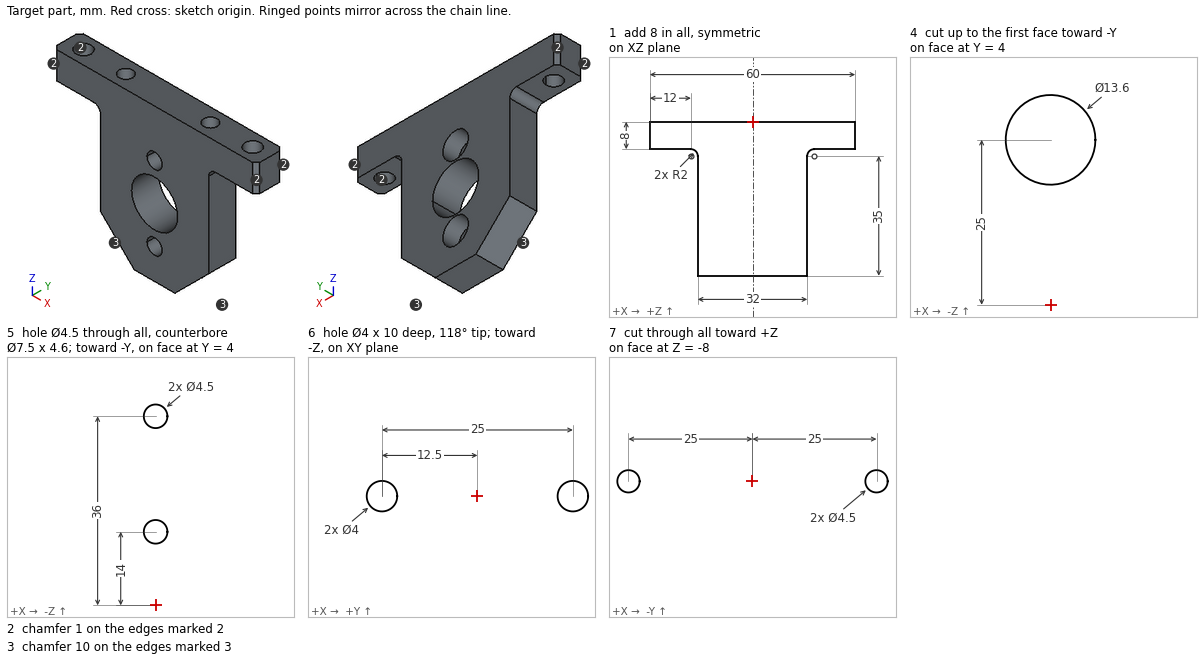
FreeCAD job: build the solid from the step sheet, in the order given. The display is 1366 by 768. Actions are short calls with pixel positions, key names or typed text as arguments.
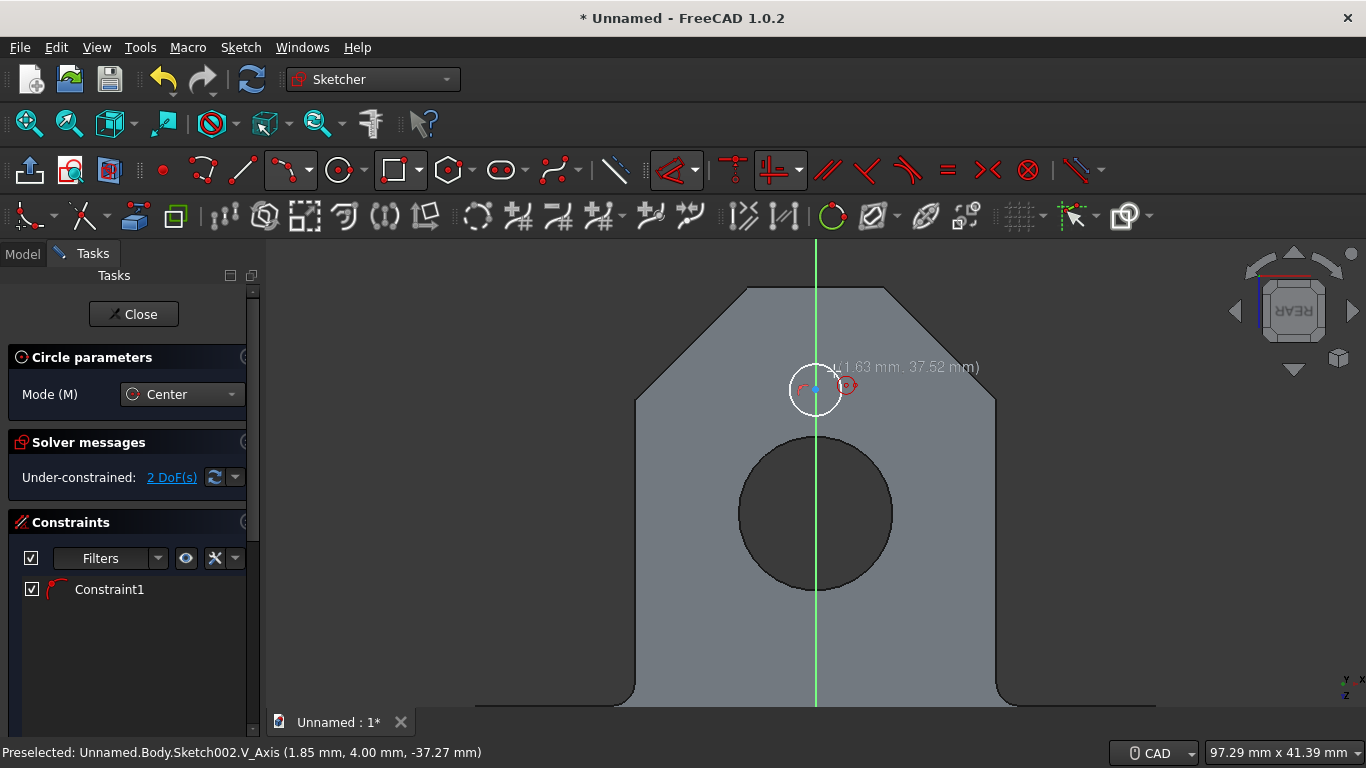
click(816, 638)
click(834, 620)
key(Escape)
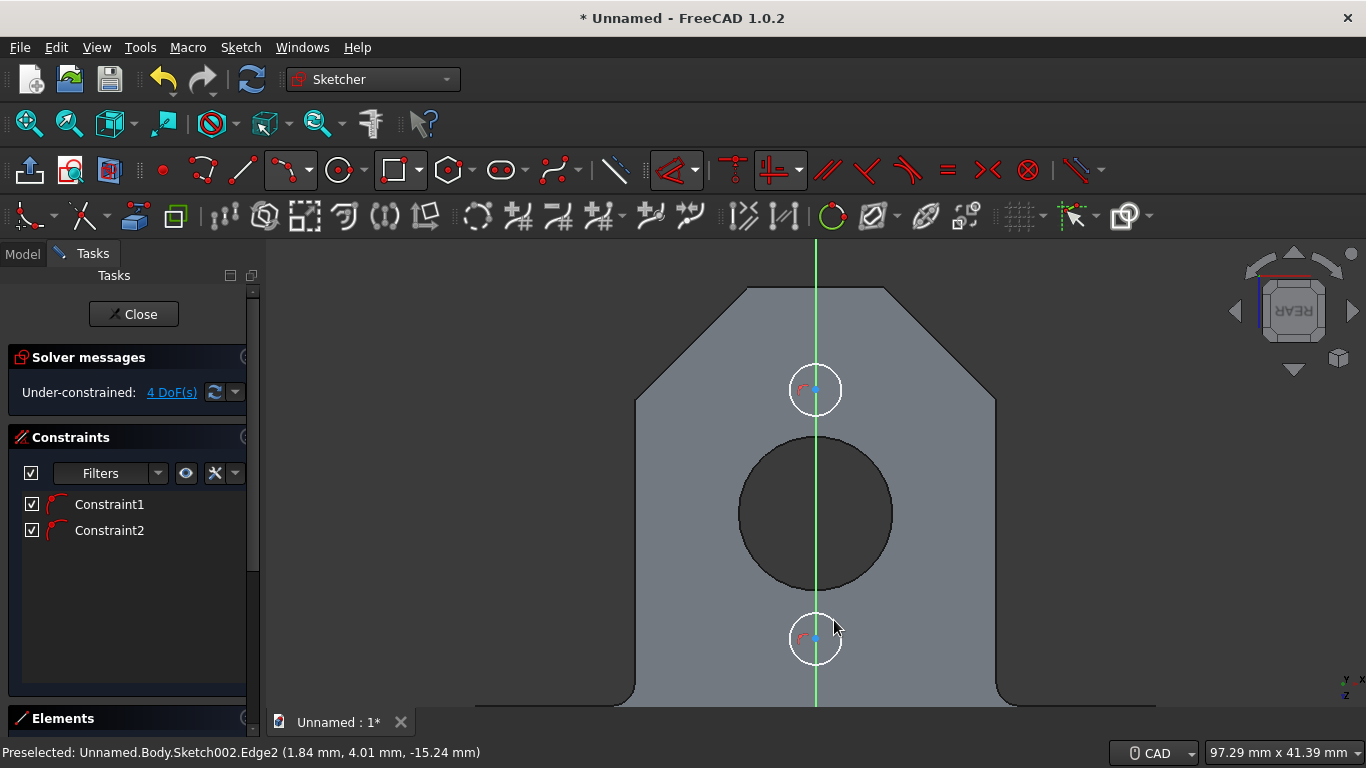
click(834, 372)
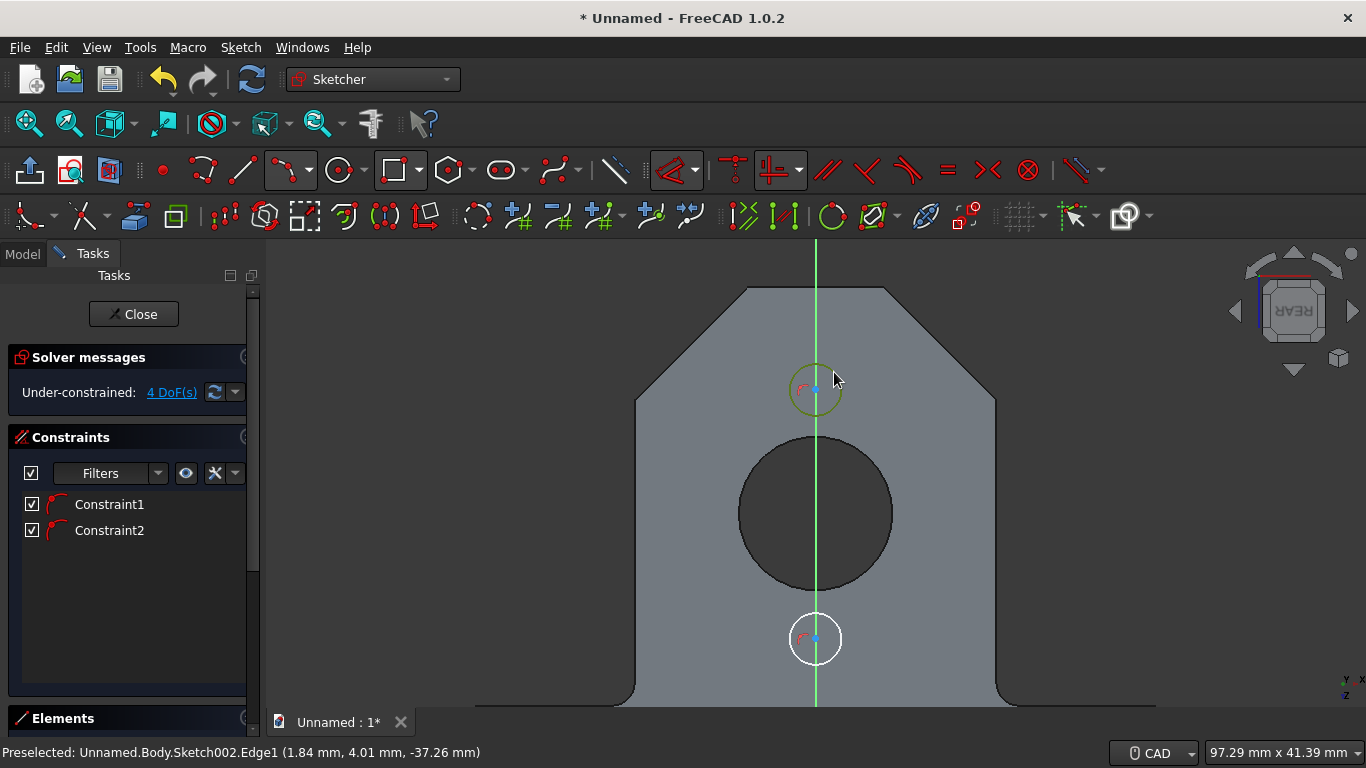
click(834, 621)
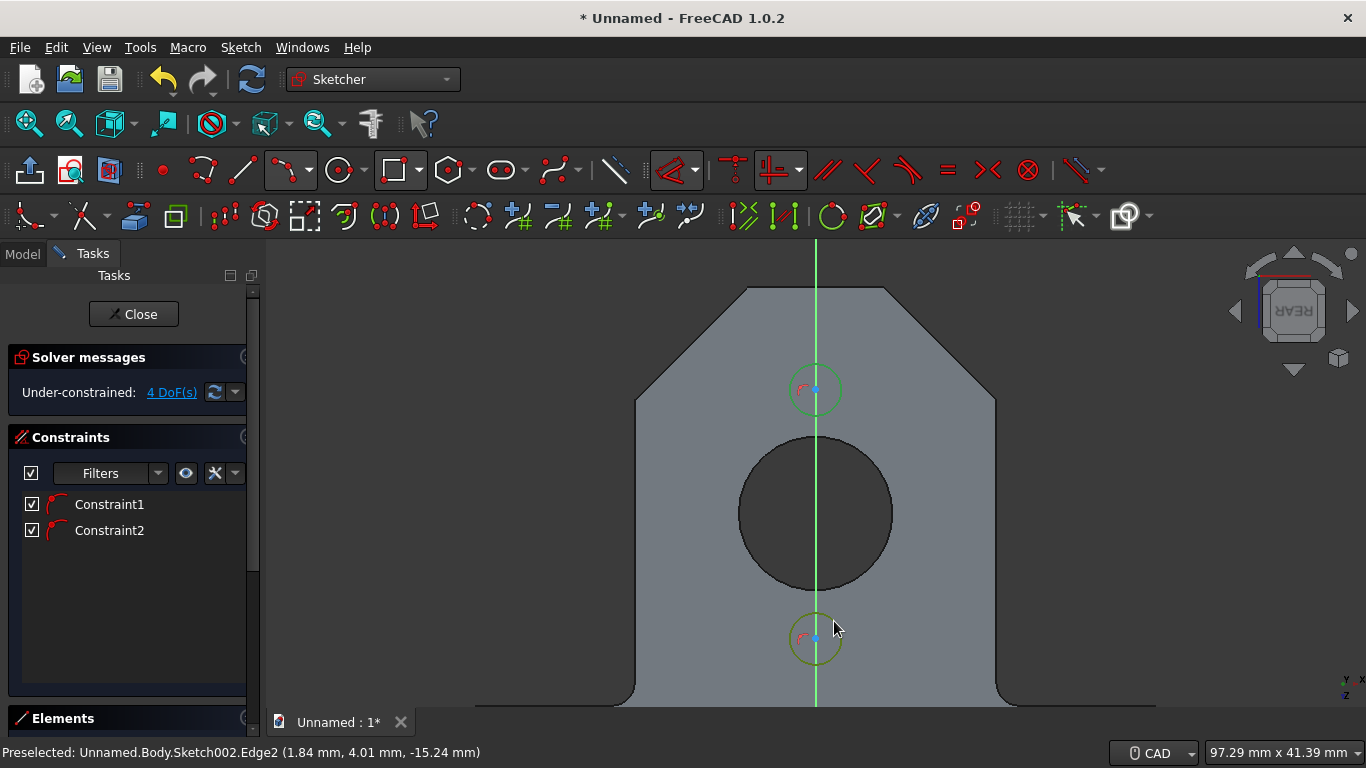
click(948, 170)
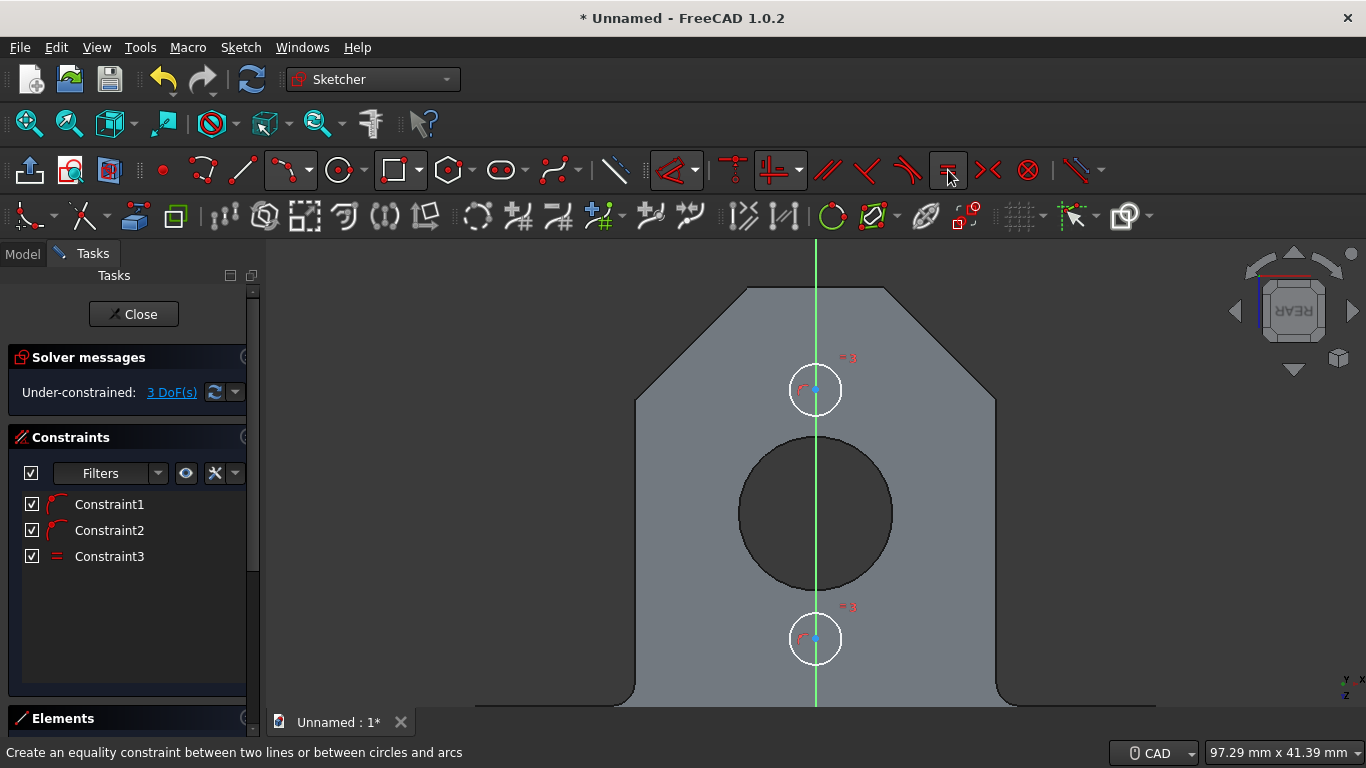
click(834, 372)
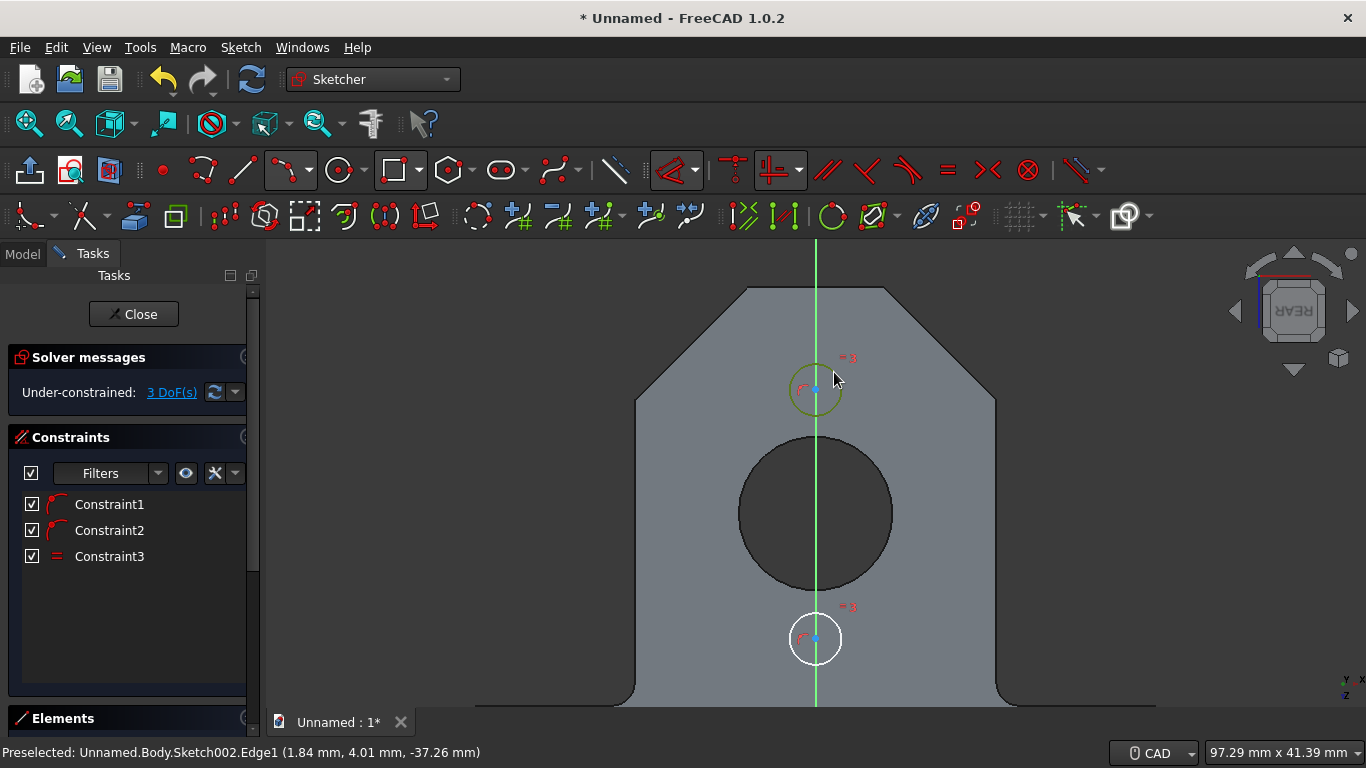
click(698, 170)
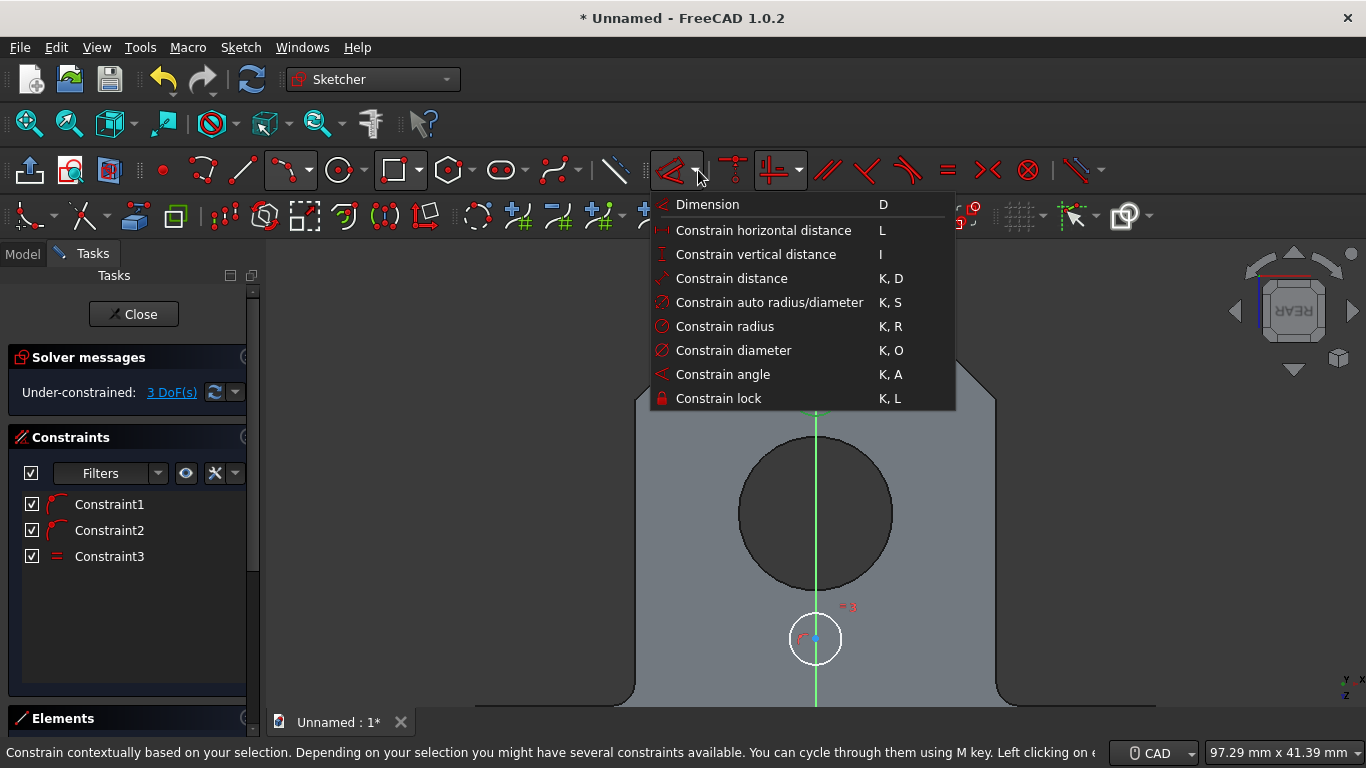
click(803, 350)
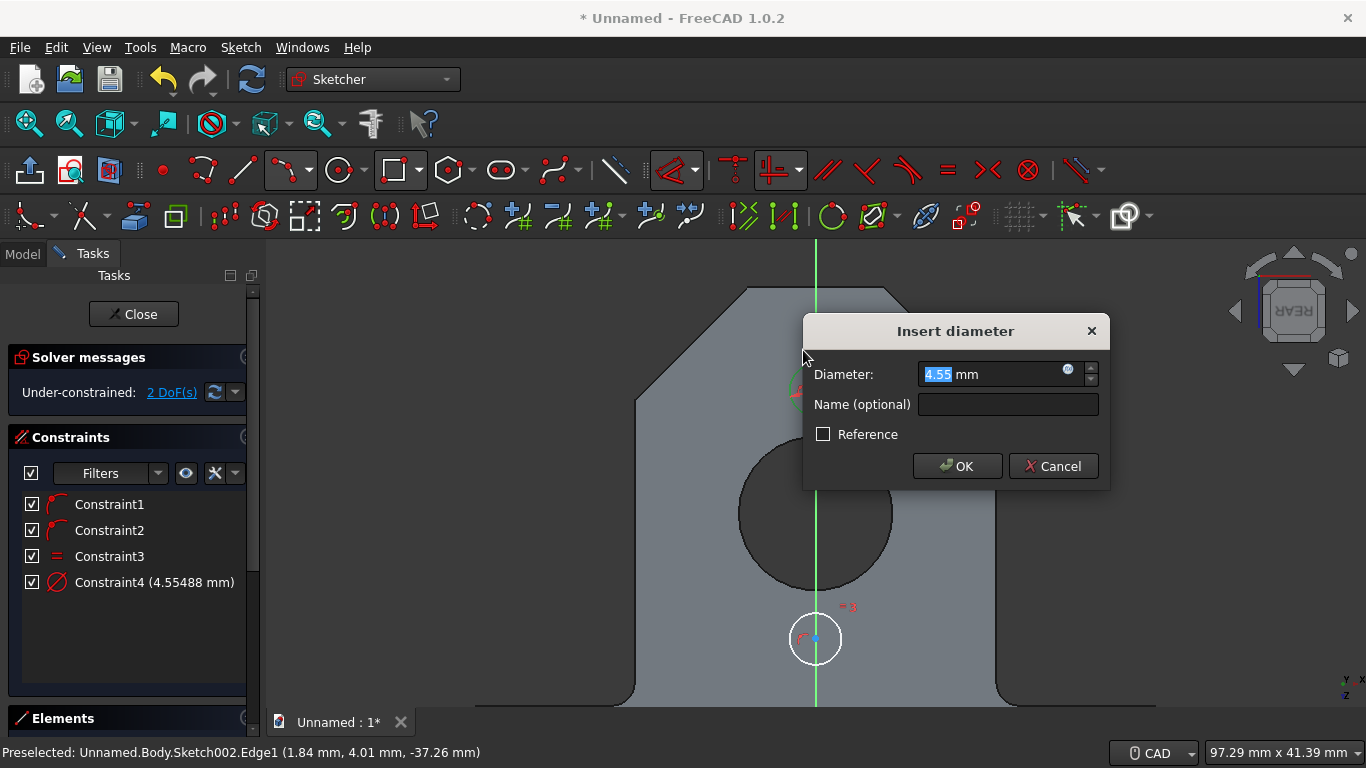
text(4.5)
key(Return)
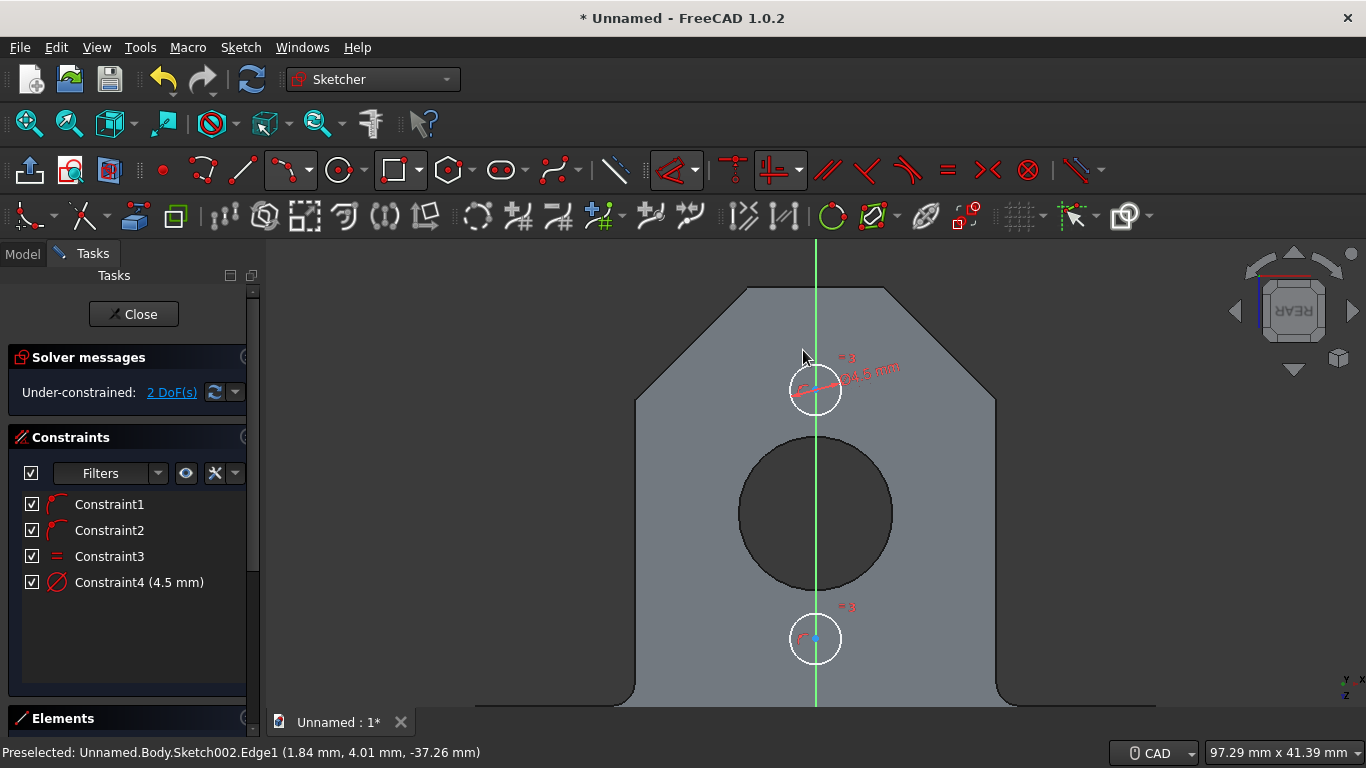
click(816, 390)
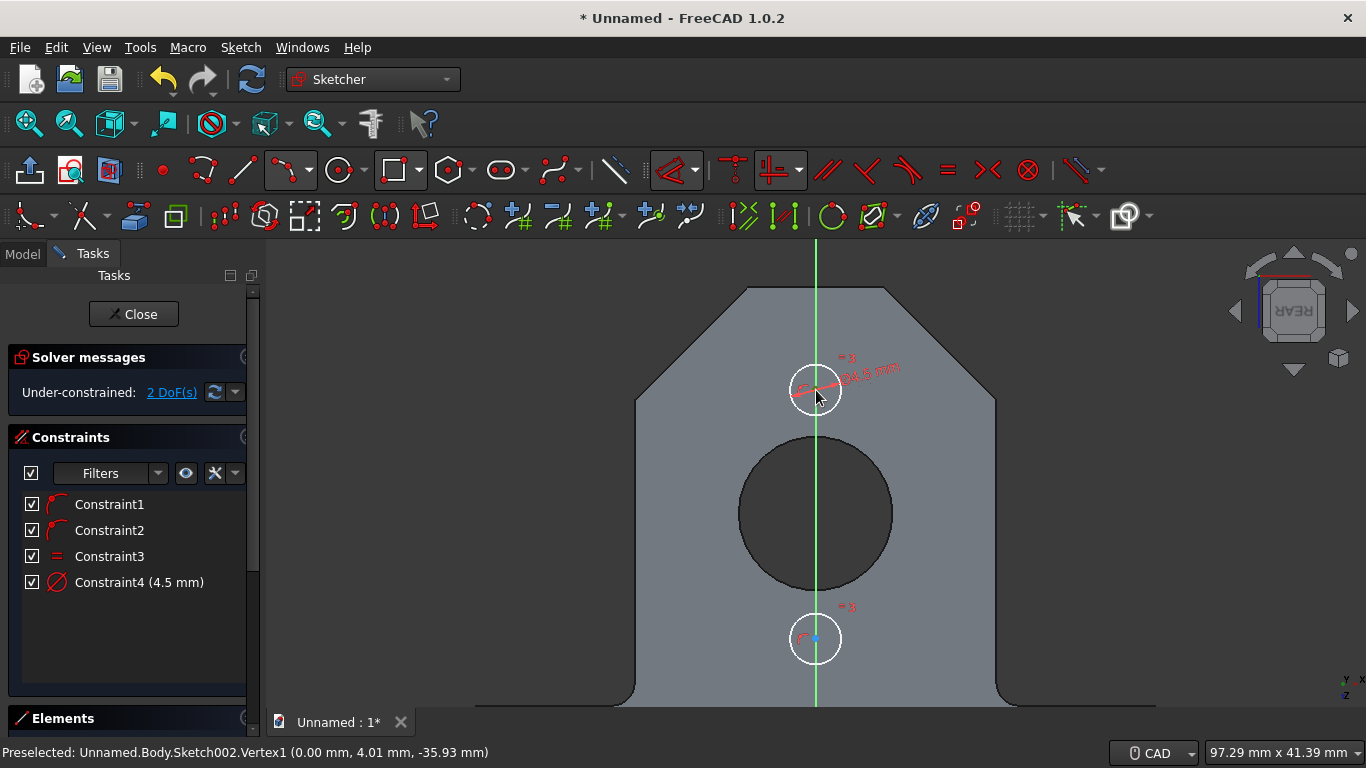
click(698, 170)